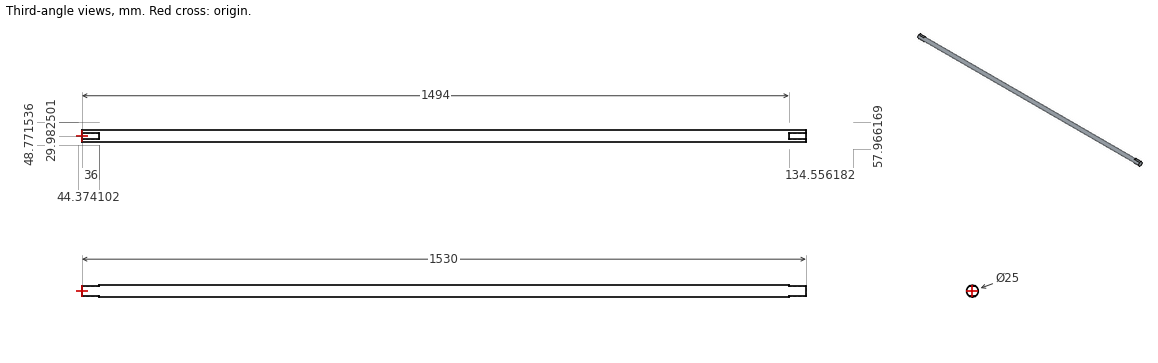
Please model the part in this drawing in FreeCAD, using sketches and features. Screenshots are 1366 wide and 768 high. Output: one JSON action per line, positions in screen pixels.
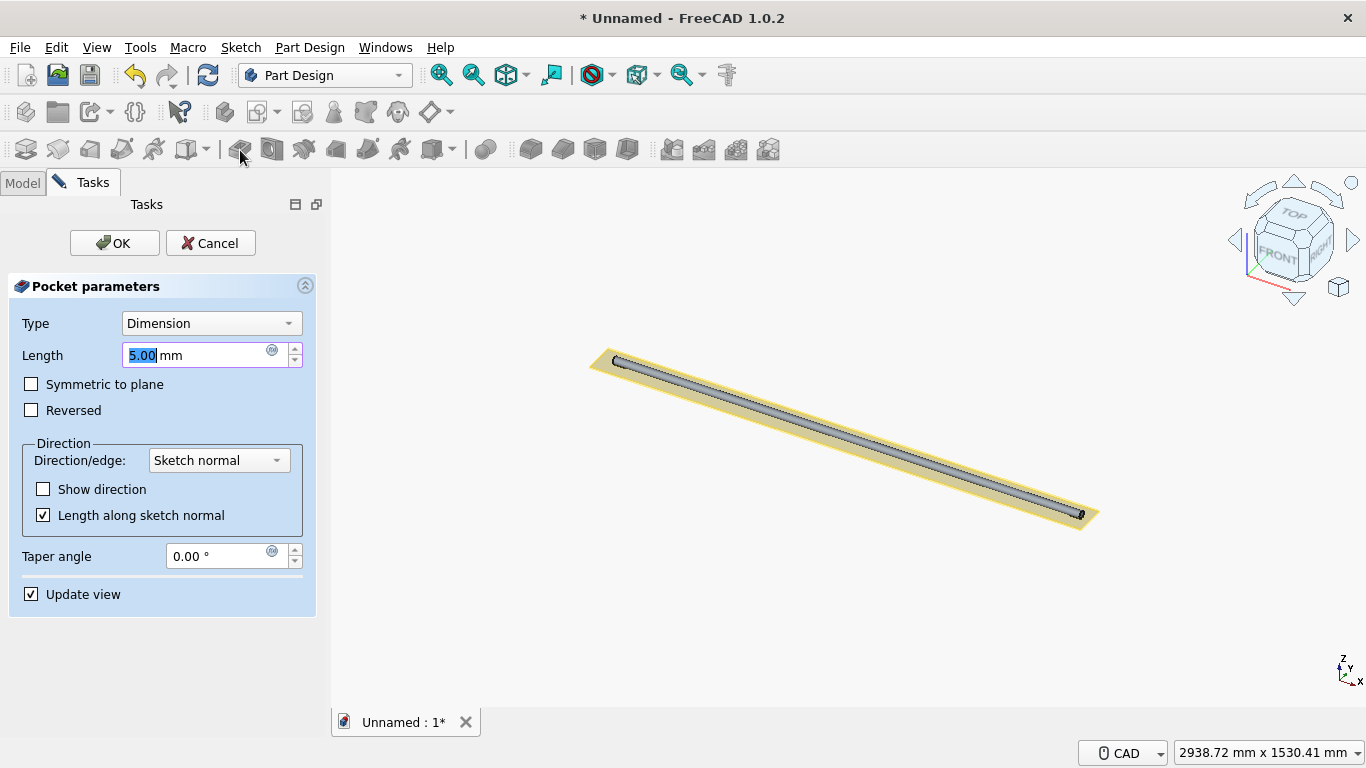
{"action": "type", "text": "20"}
{"action": "key", "text": "Tab"}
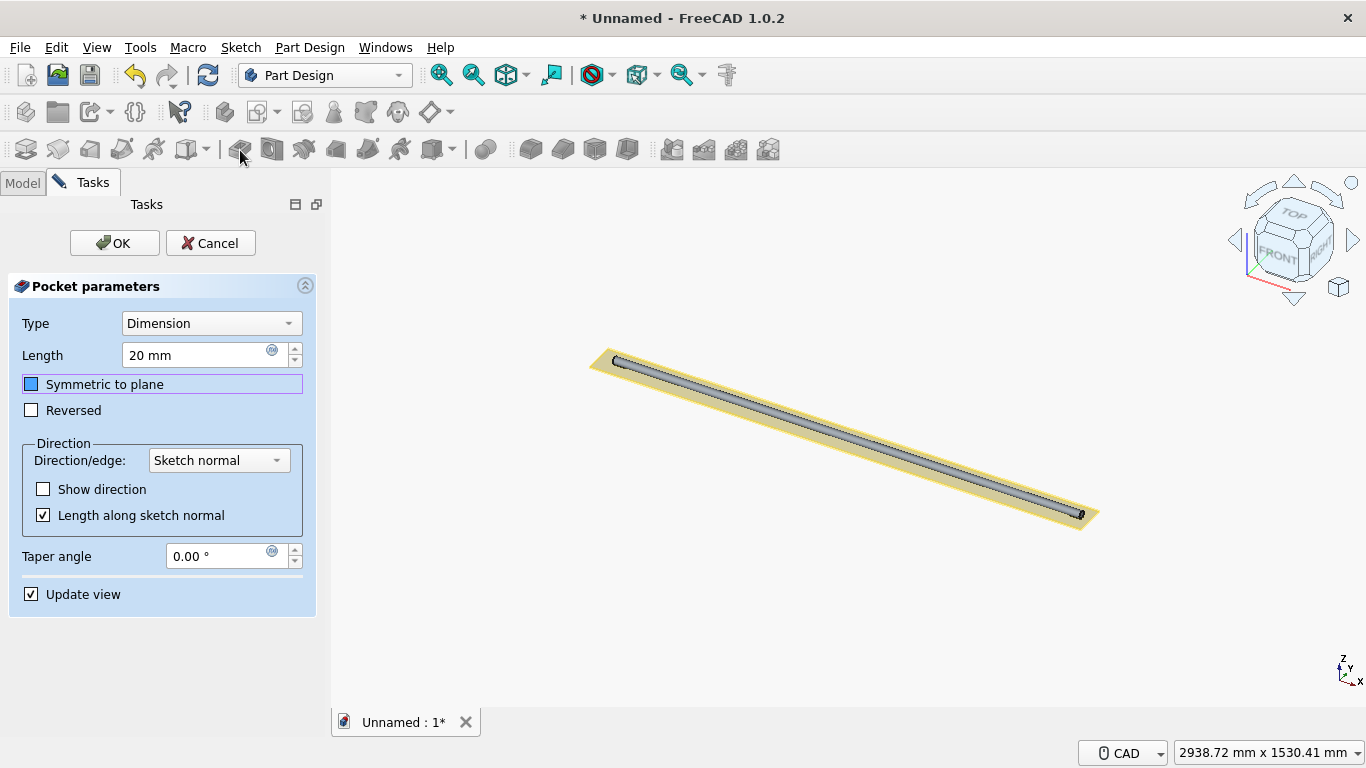
{"action": "left_click", "coordinate": [115, 243]}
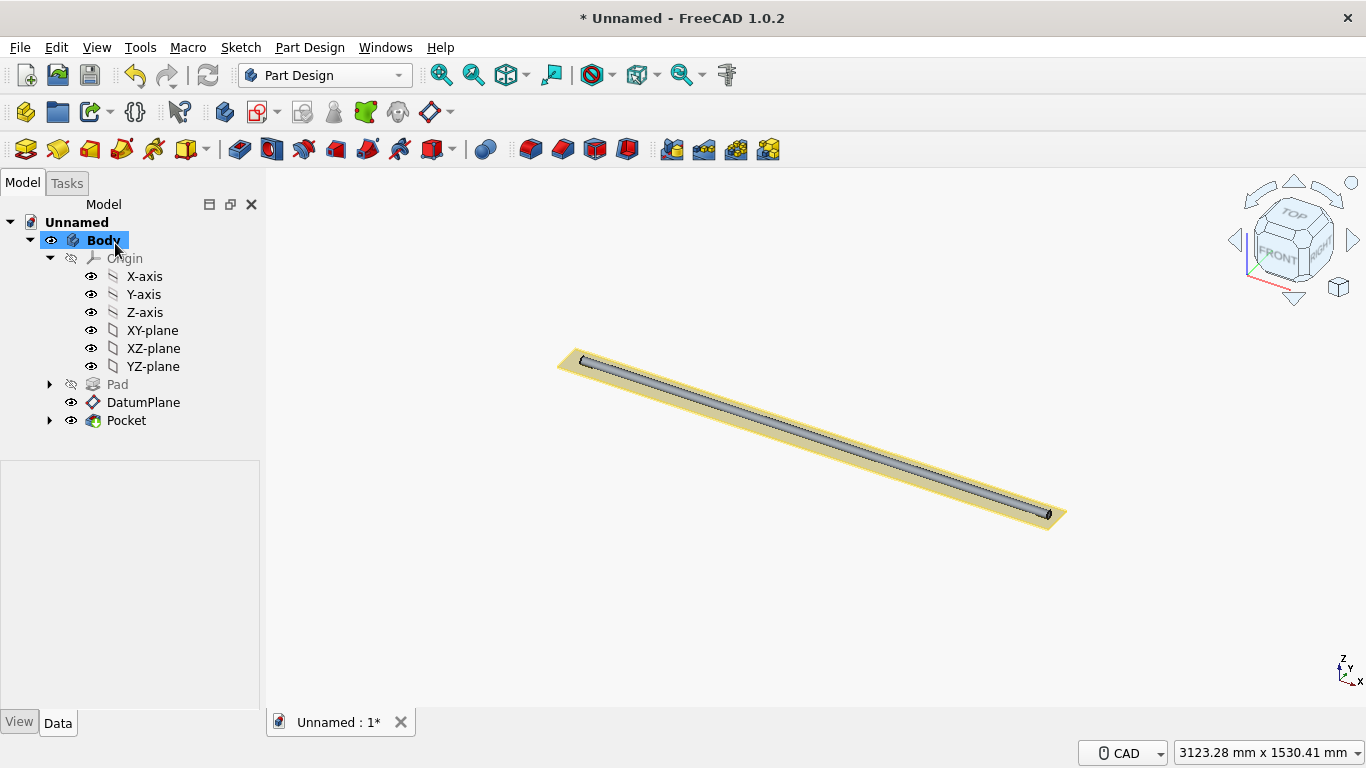
{"action": "left_click", "coordinate": [116, 402]}
{"action": "key", "text": "space"}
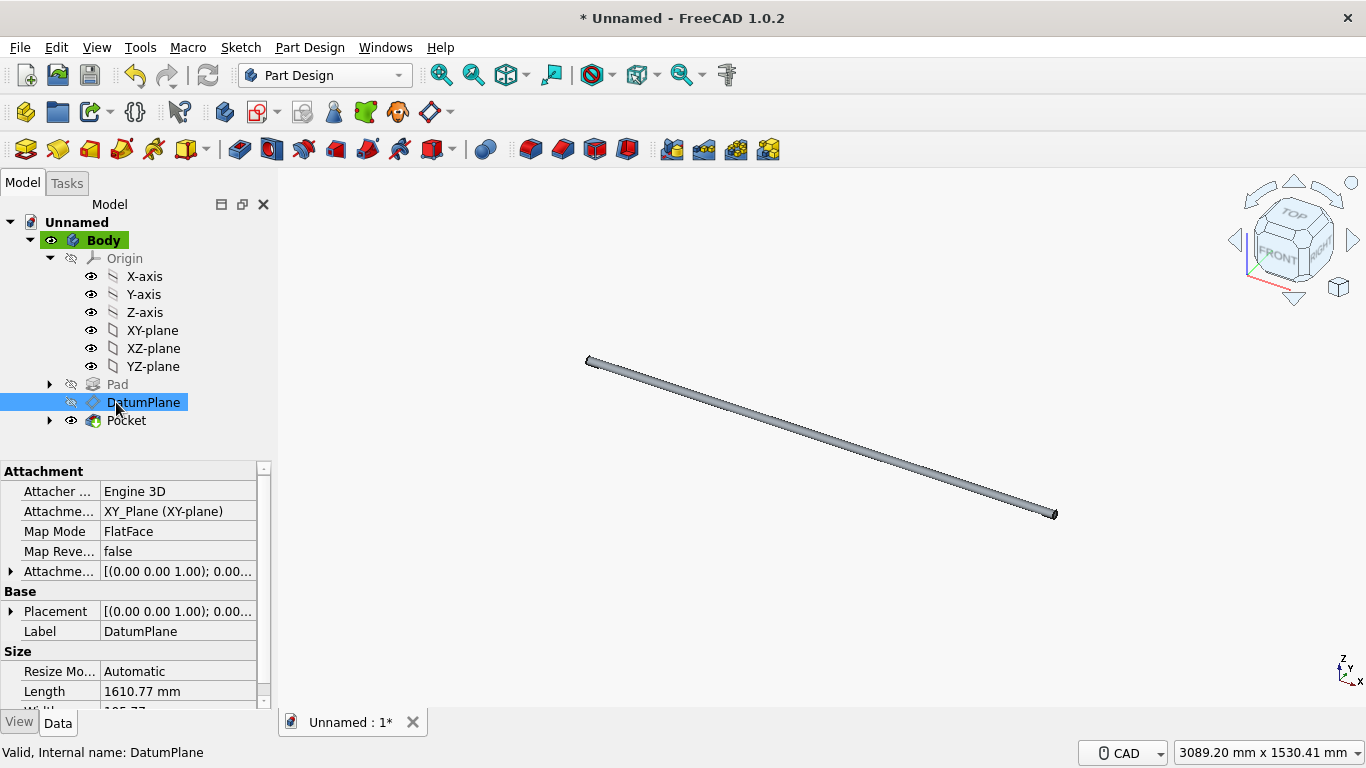
{"action": "left_click", "coordinate": [442, 76]}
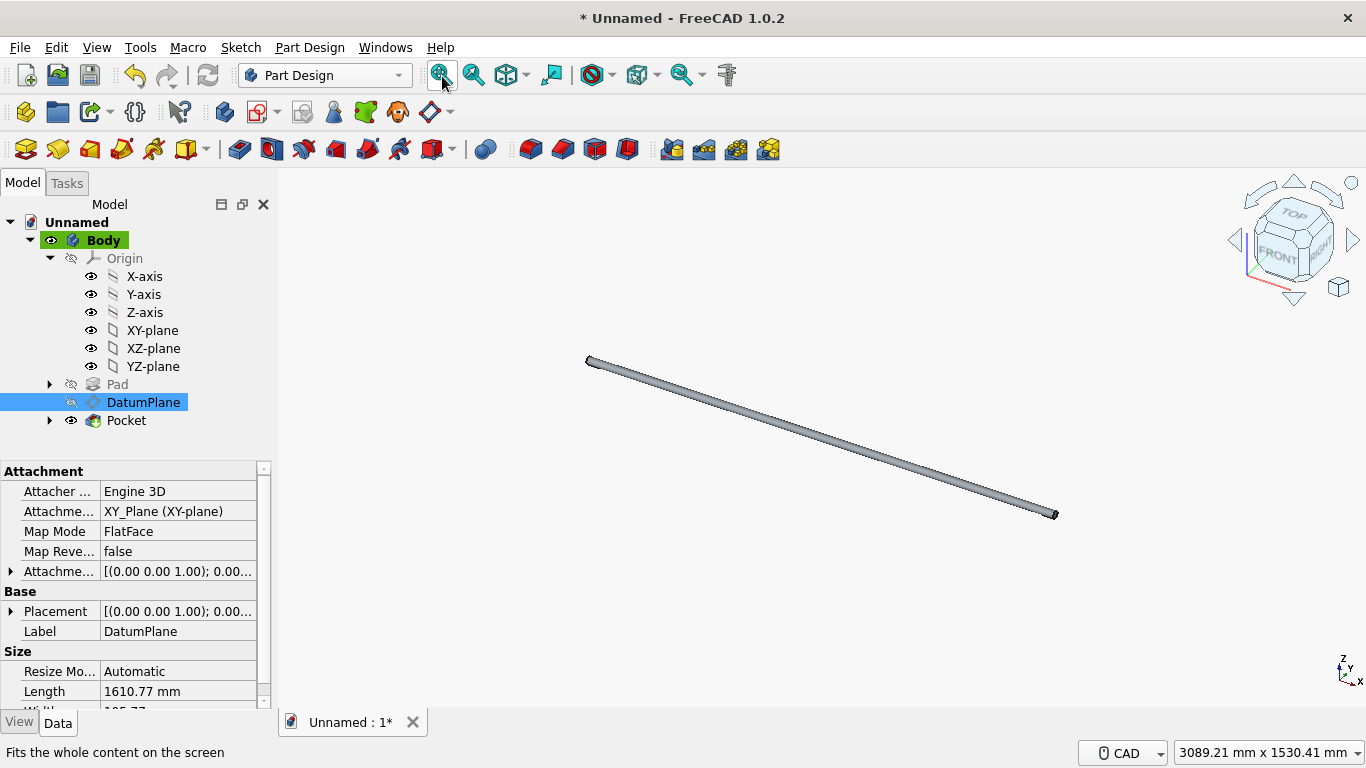
{"action": "left_click", "coordinate": [136, 330]}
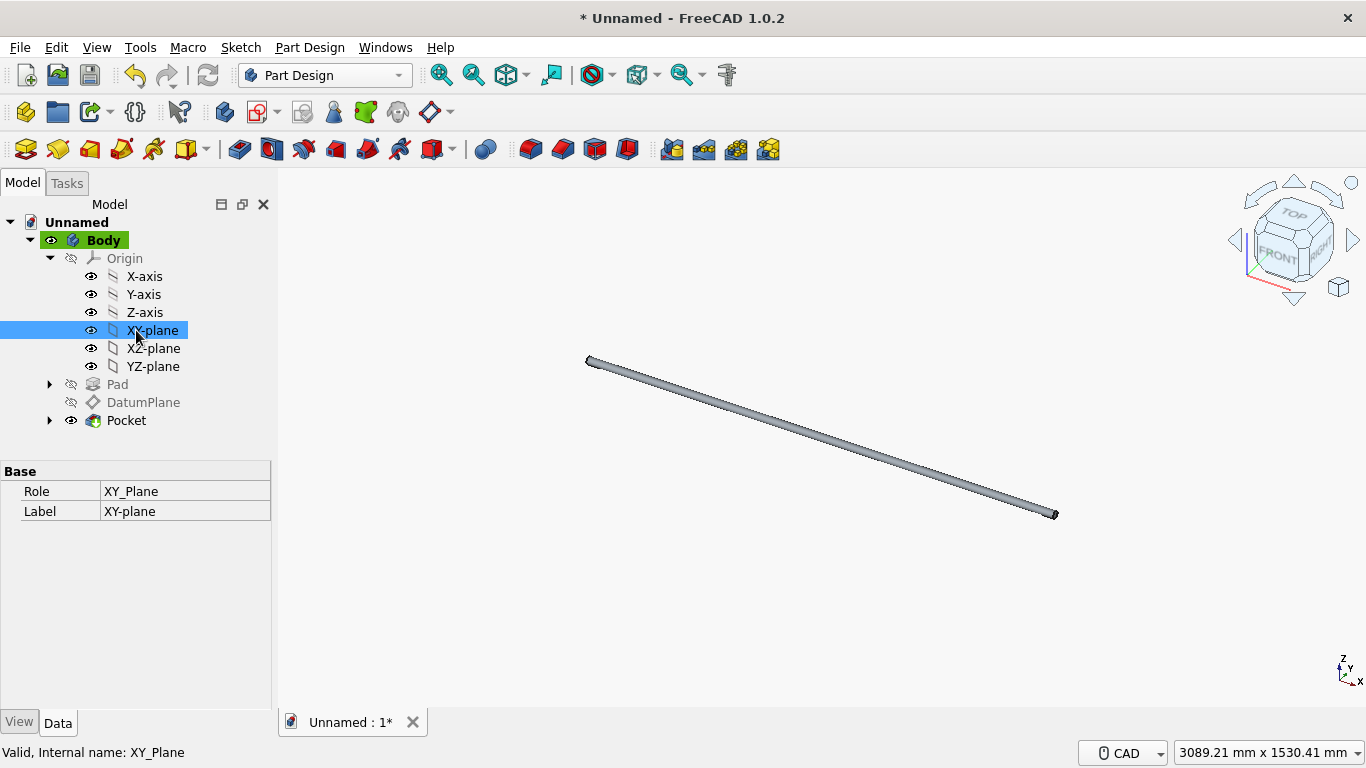
{"action": "left_click", "coordinate": [430, 112]}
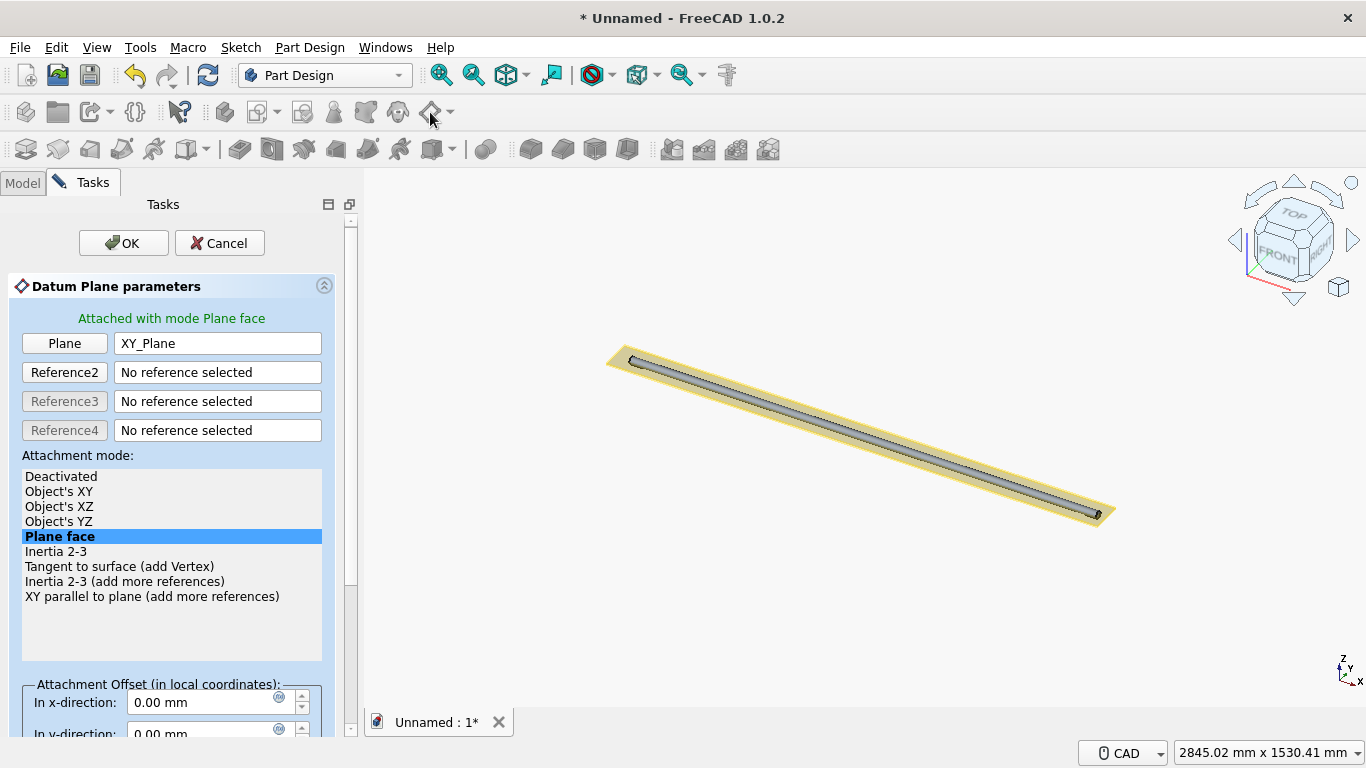
{"action": "scroll", "coordinate": [351, 475], "scroll_direction": "down", "scroll_amount": 2}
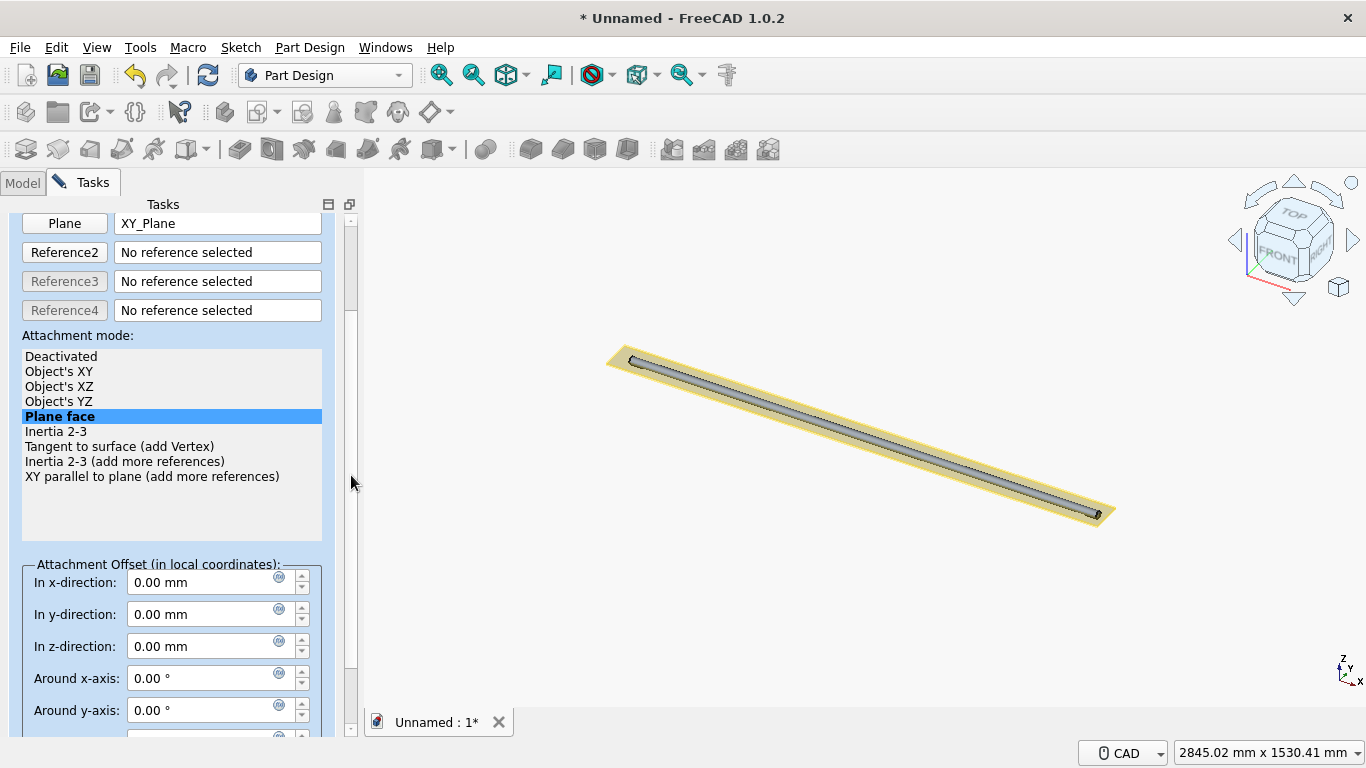
{"action": "triple_click", "coordinate": [210, 646]}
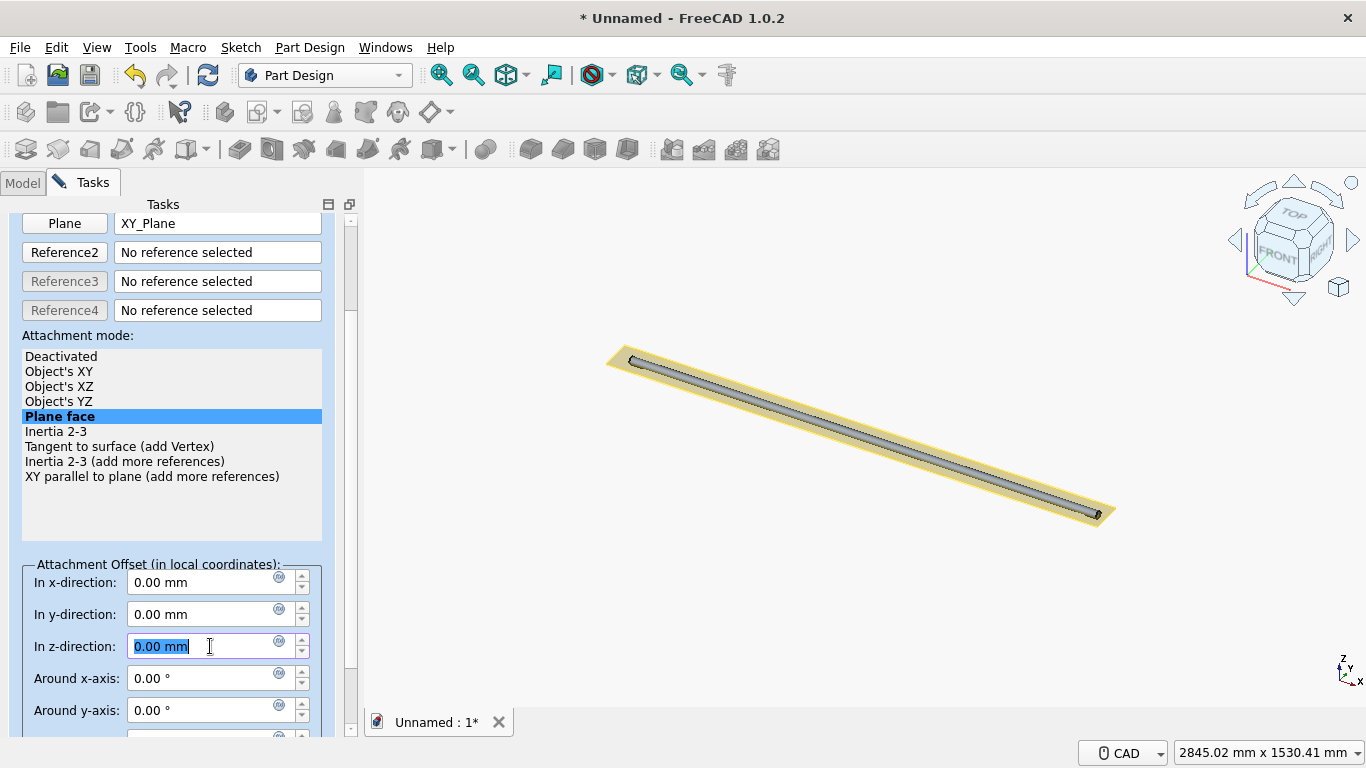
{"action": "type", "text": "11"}
{"action": "key", "text": "Tab"}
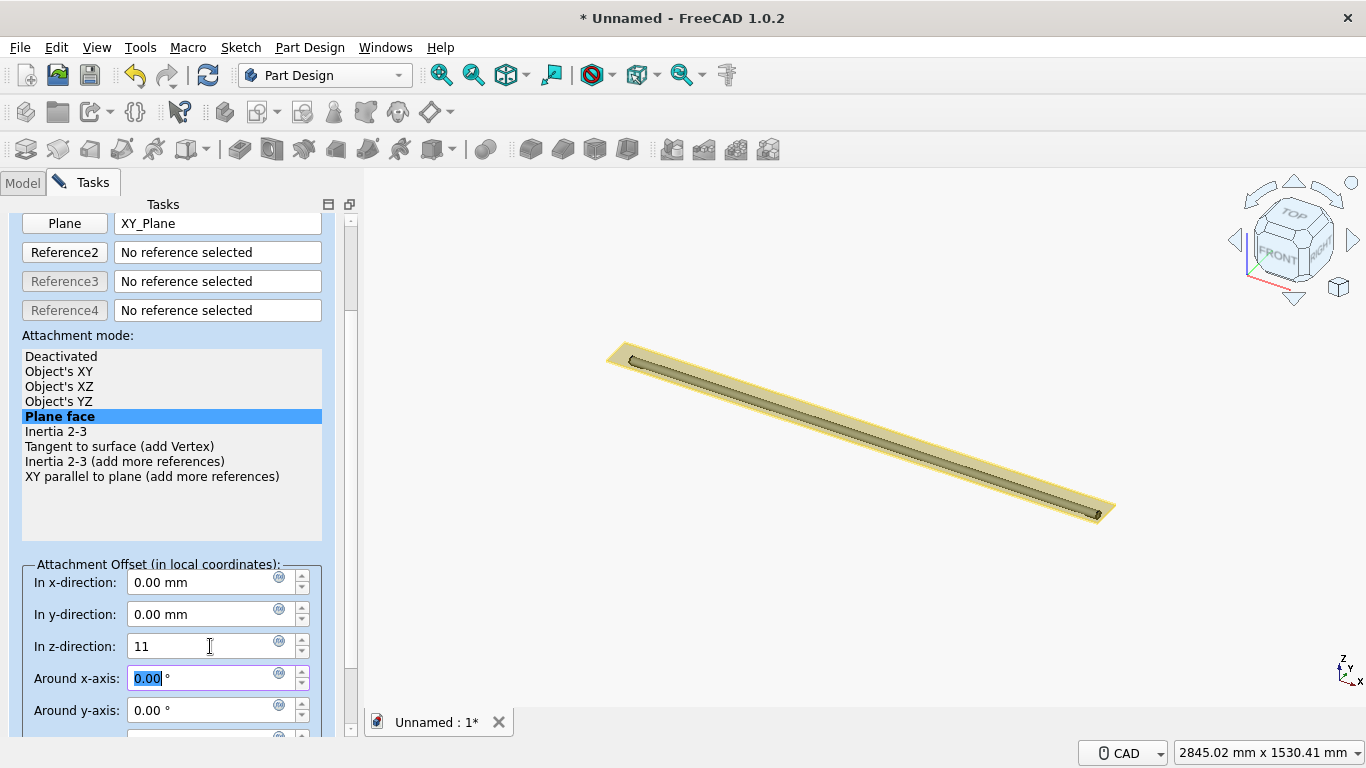
{"action": "scroll", "coordinate": [351, 475], "scroll_direction": "up", "scroll_amount": 3}